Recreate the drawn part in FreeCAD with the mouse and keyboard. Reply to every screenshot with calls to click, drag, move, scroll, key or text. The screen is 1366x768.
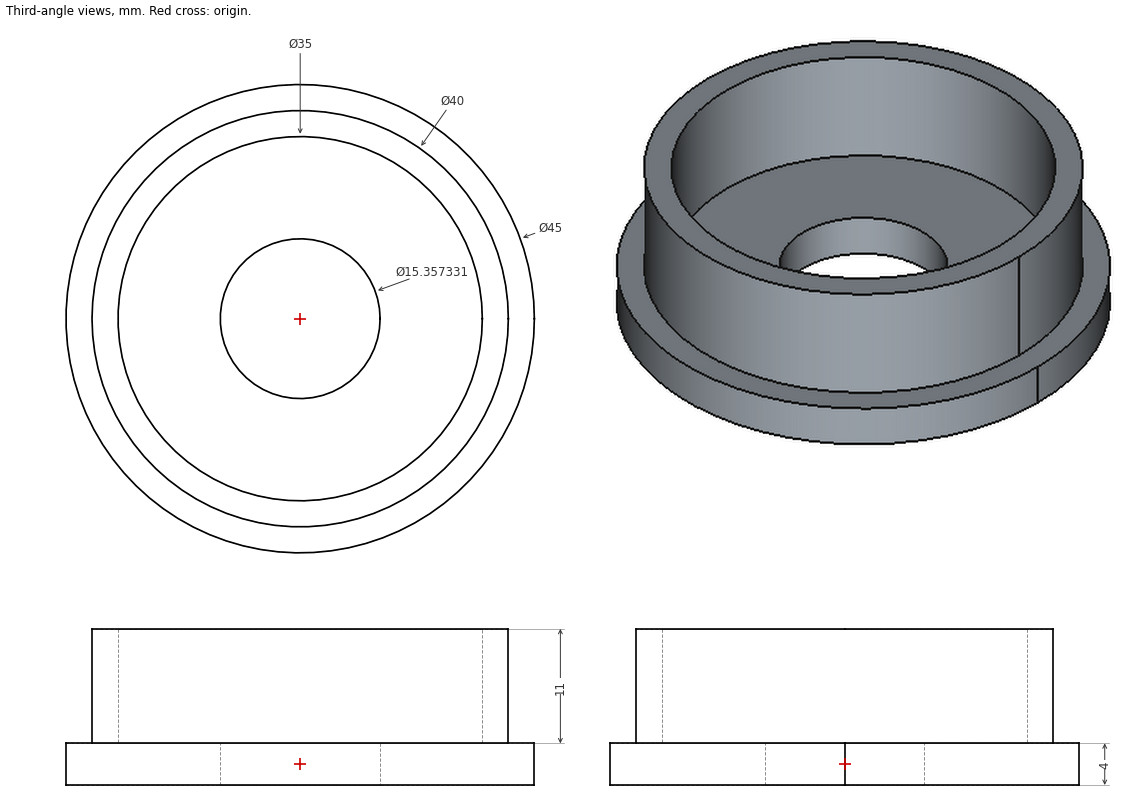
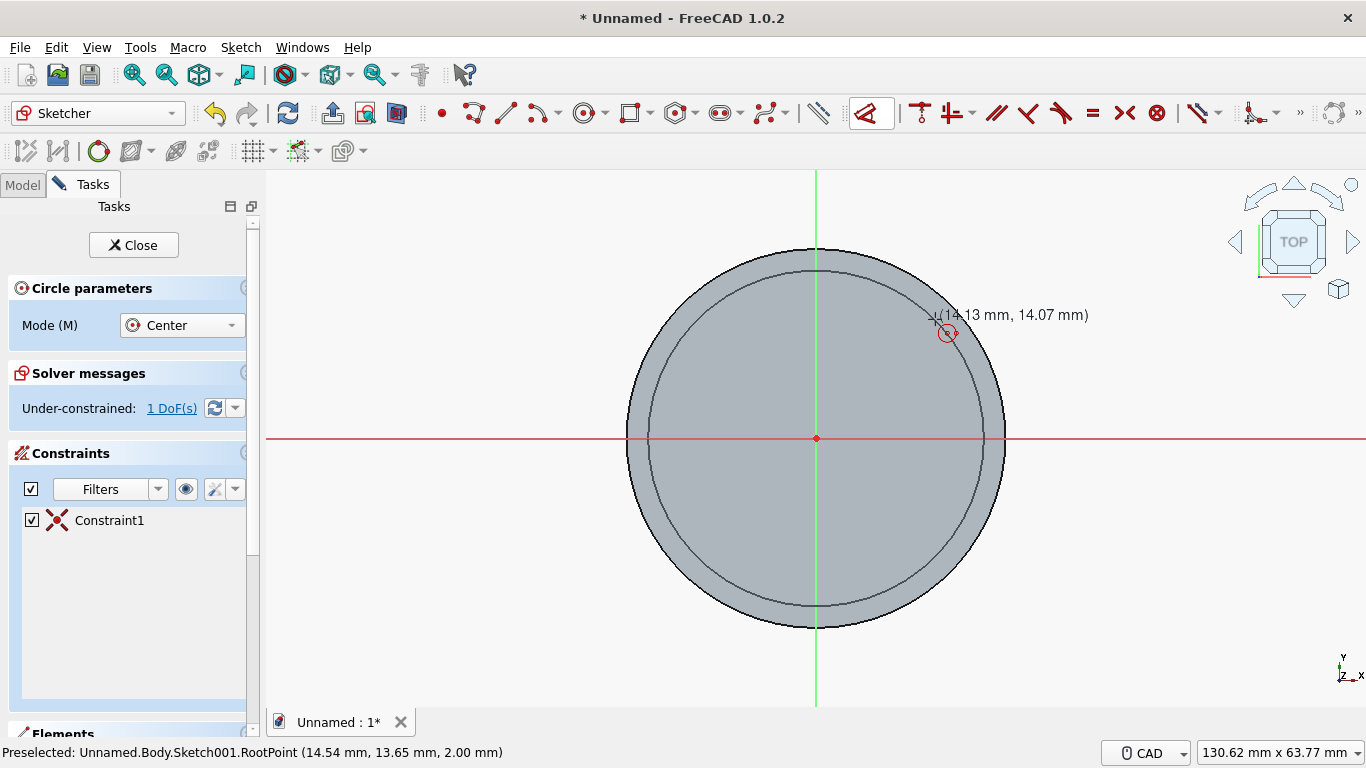
click(816, 438)
click(920, 334)
key(Escape)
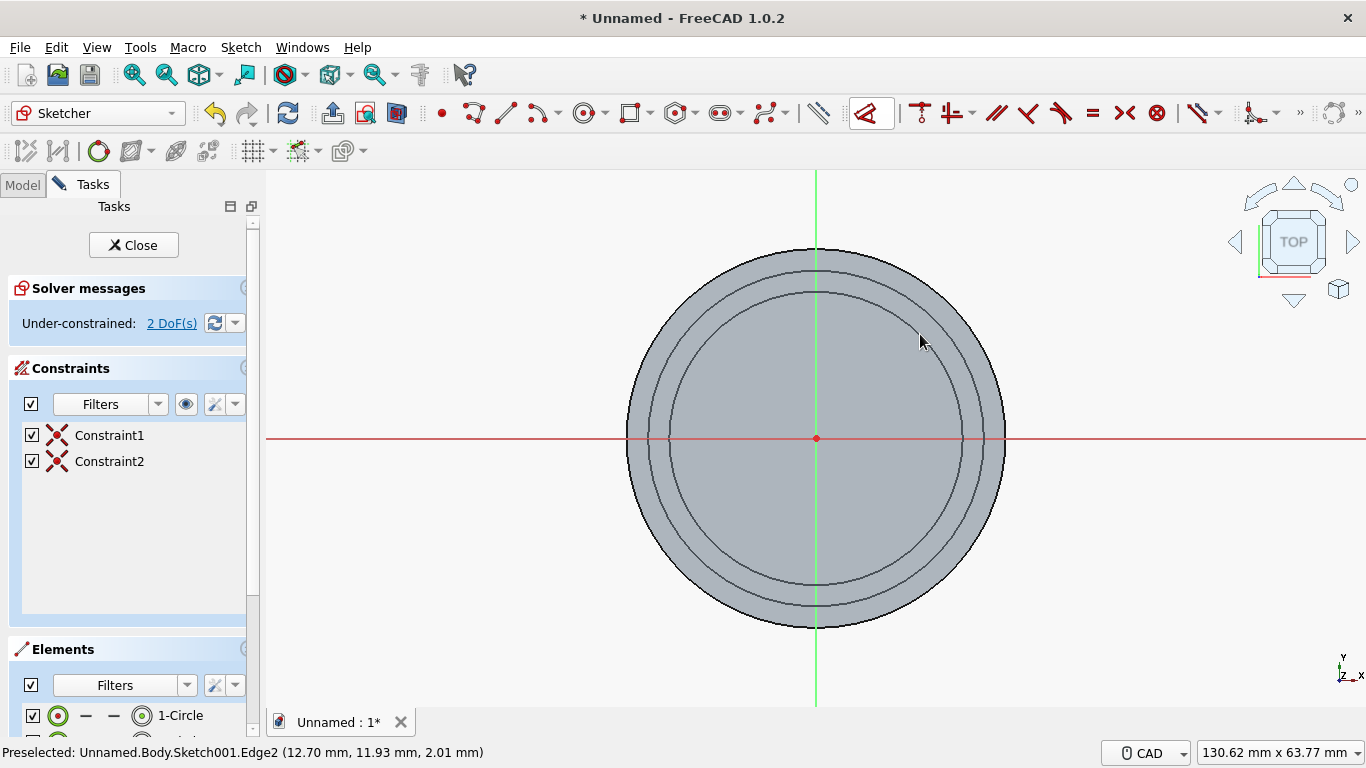
click(866, 114)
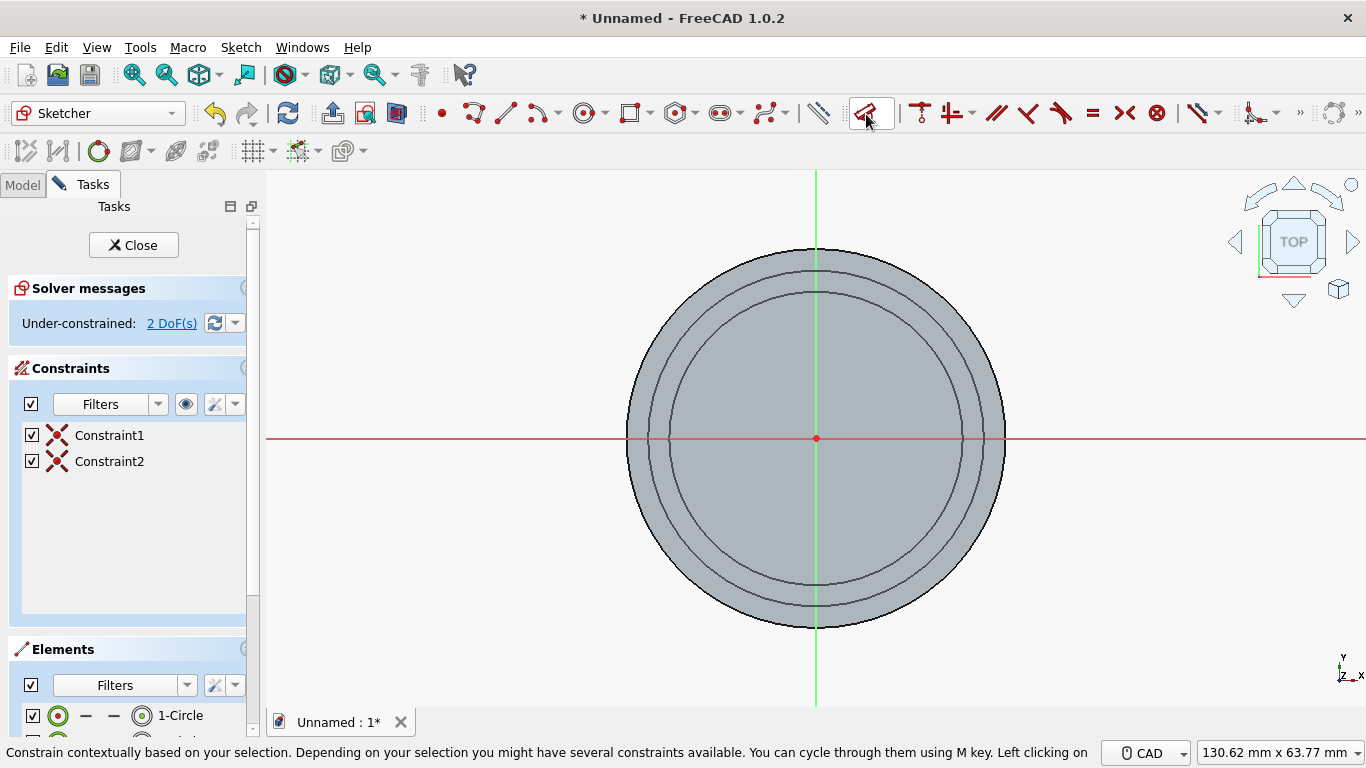
click(934, 319)
click(956, 296)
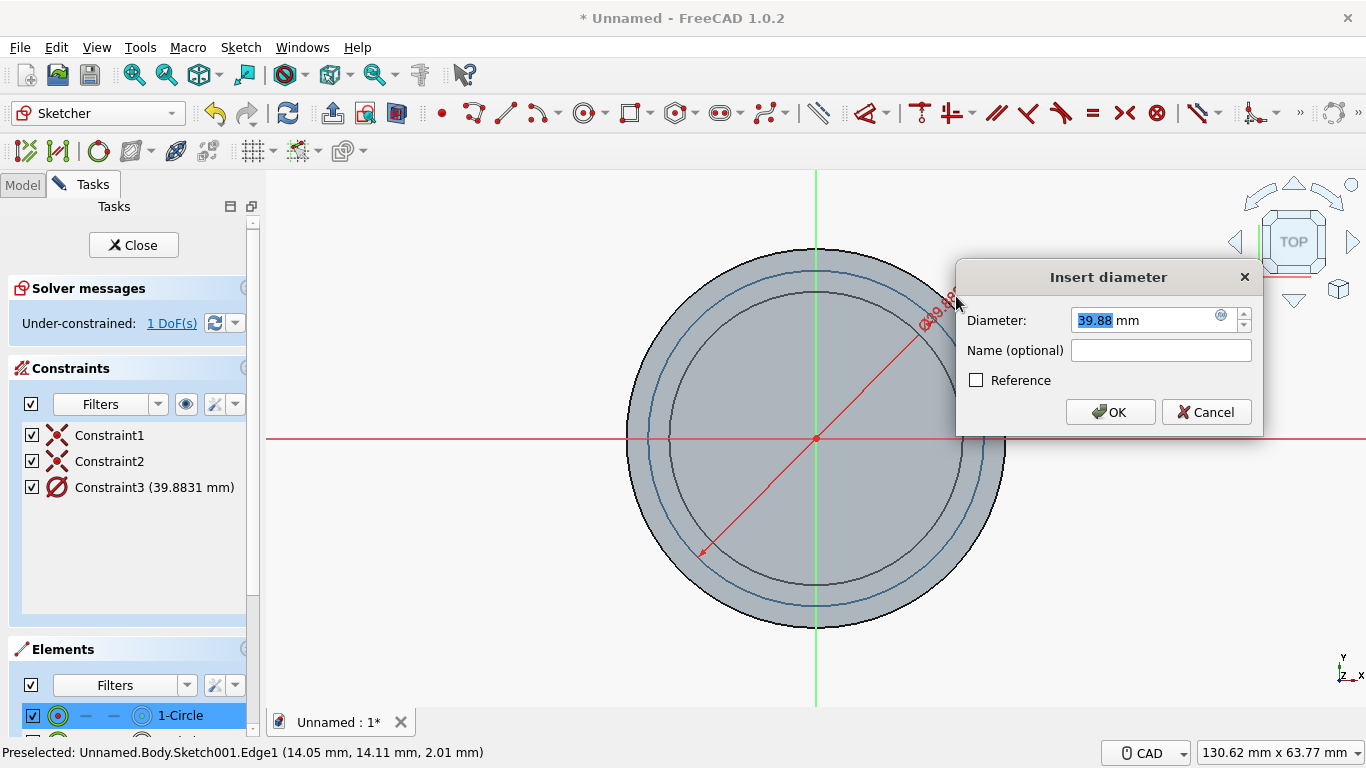
text(40)
key(Return)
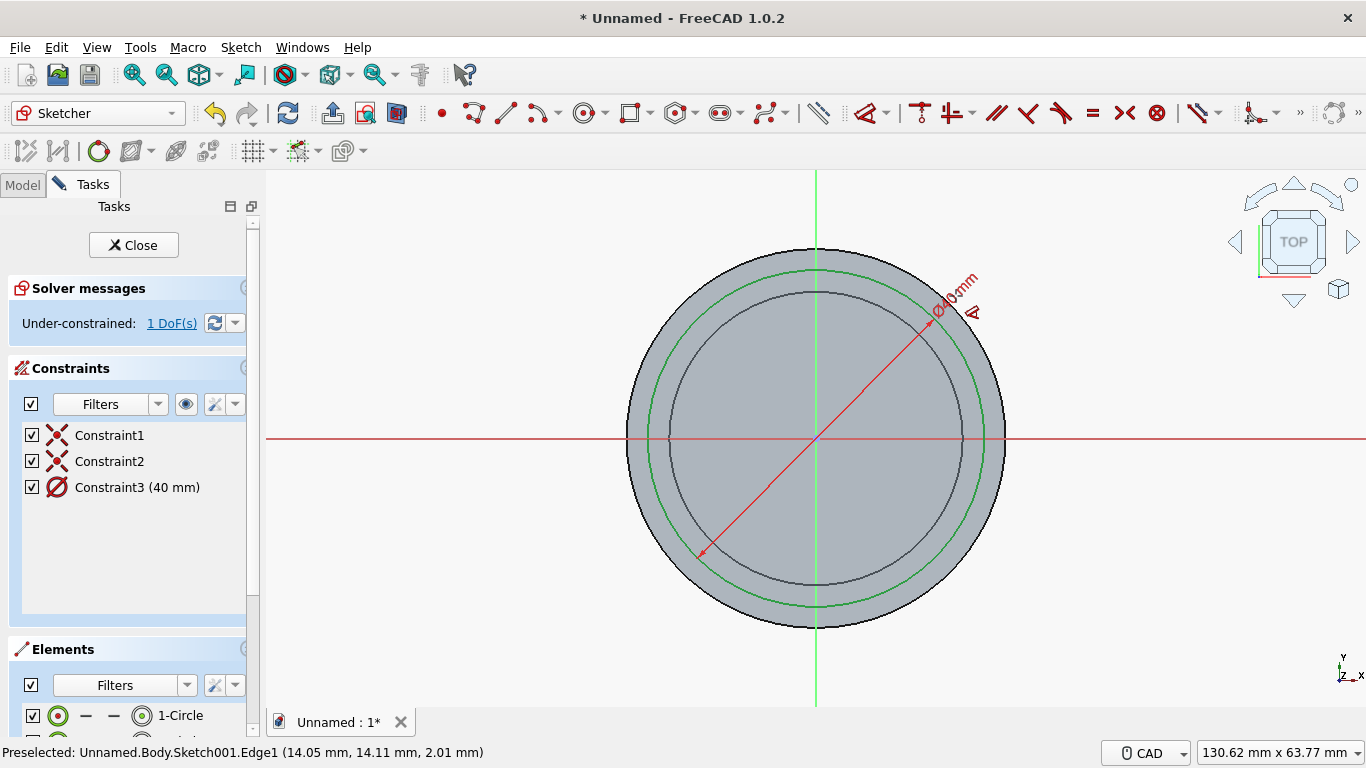
click(919, 334)
click(1009, 380)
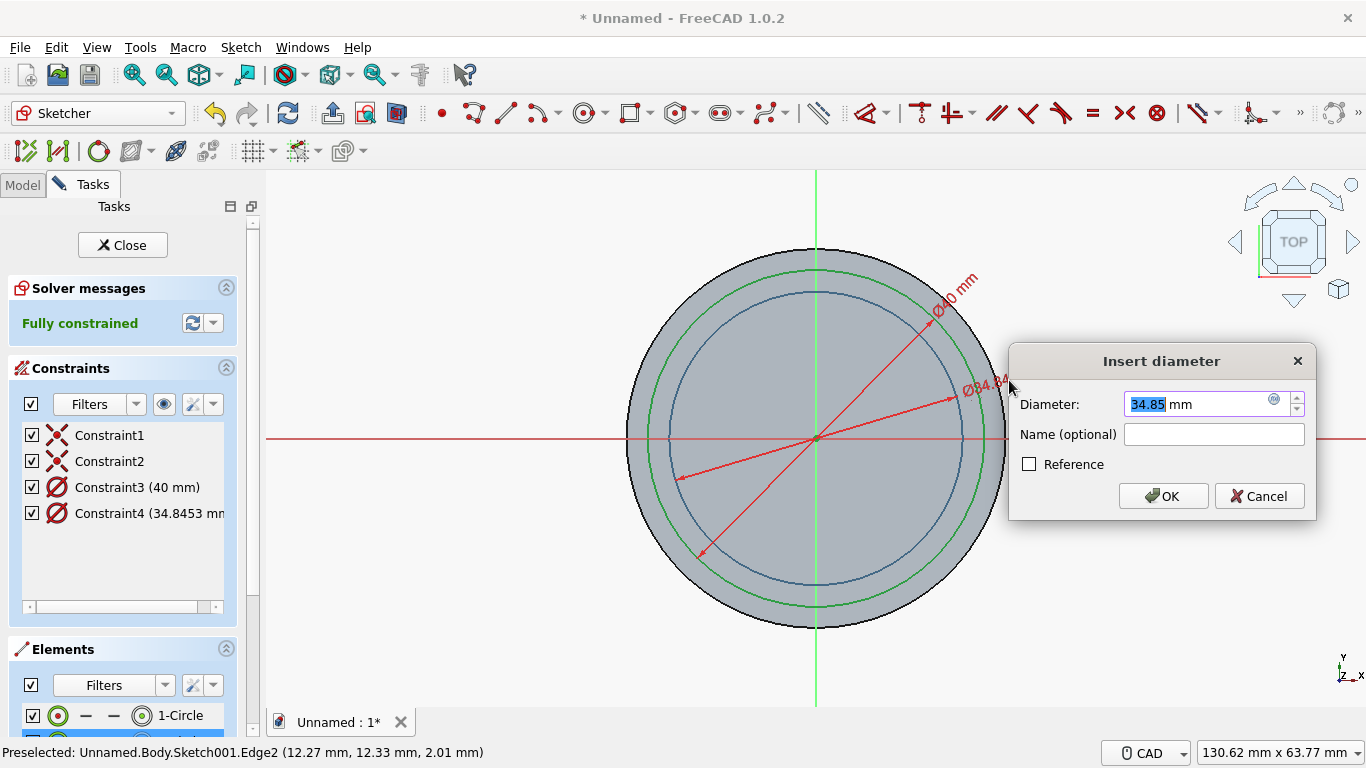
text(35)
key(Return)
key(Escape)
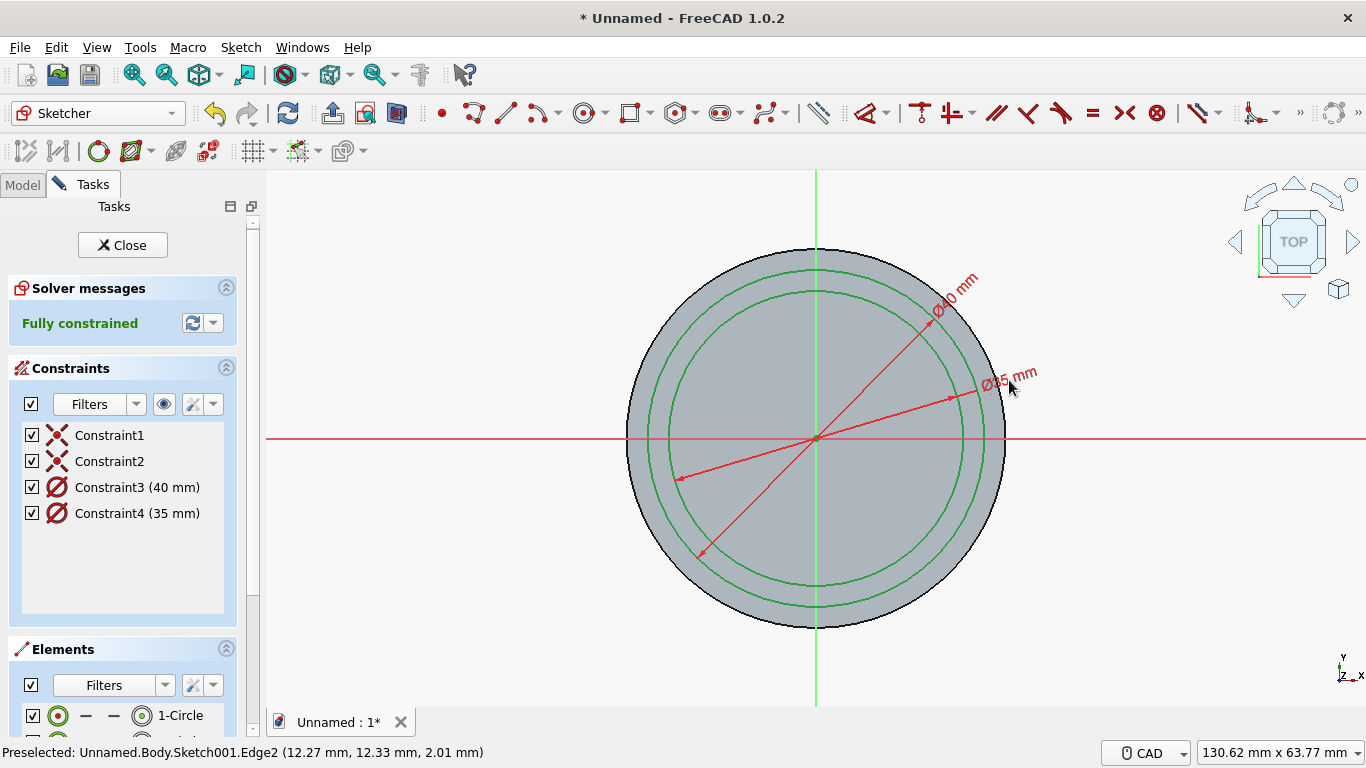
click(123, 245)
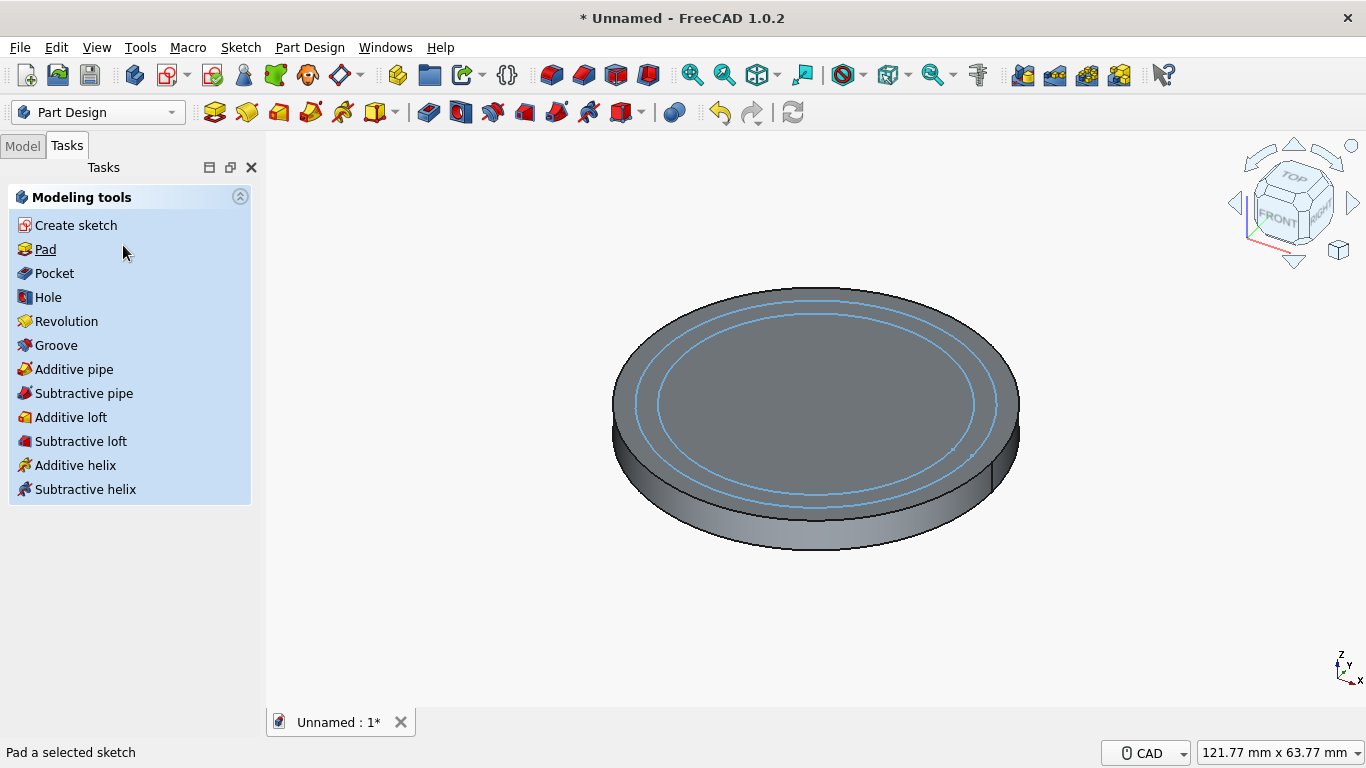
click(216, 112)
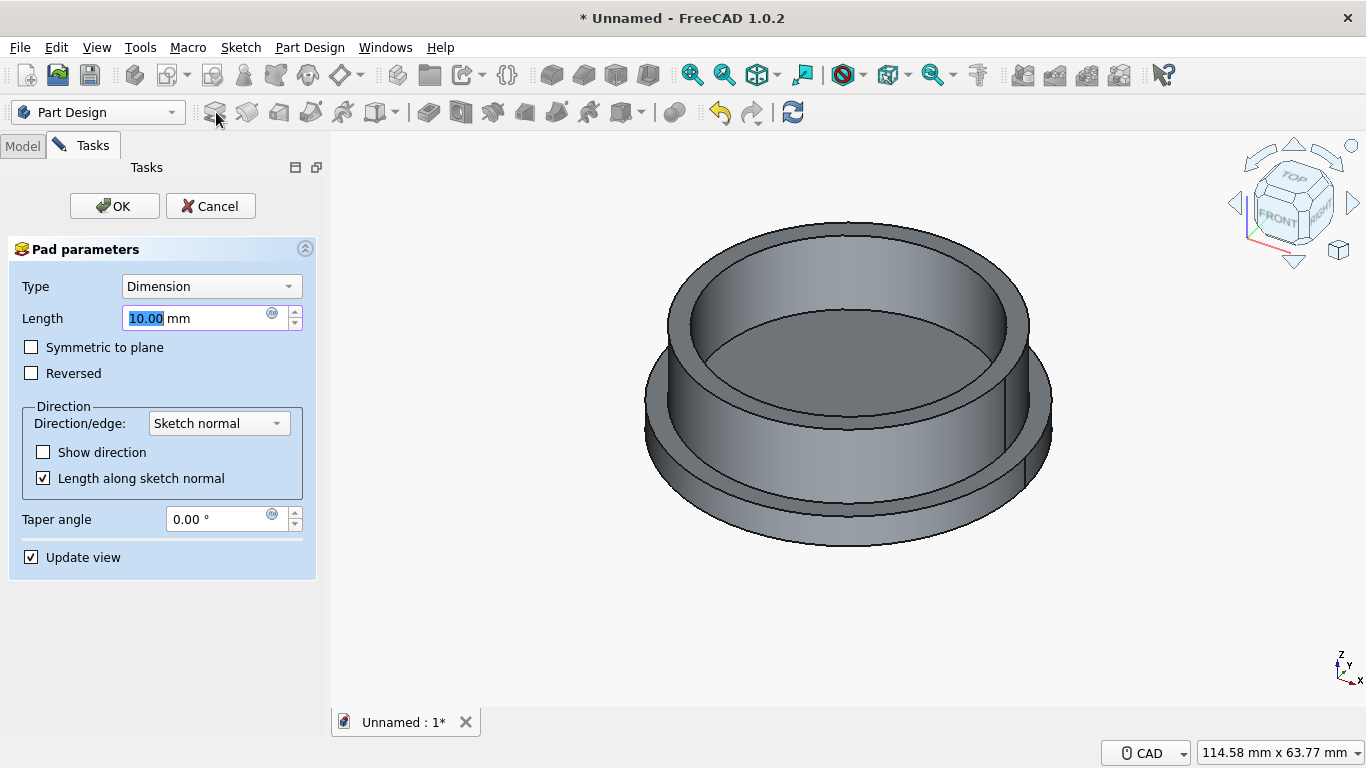
text(11)
key(Tab)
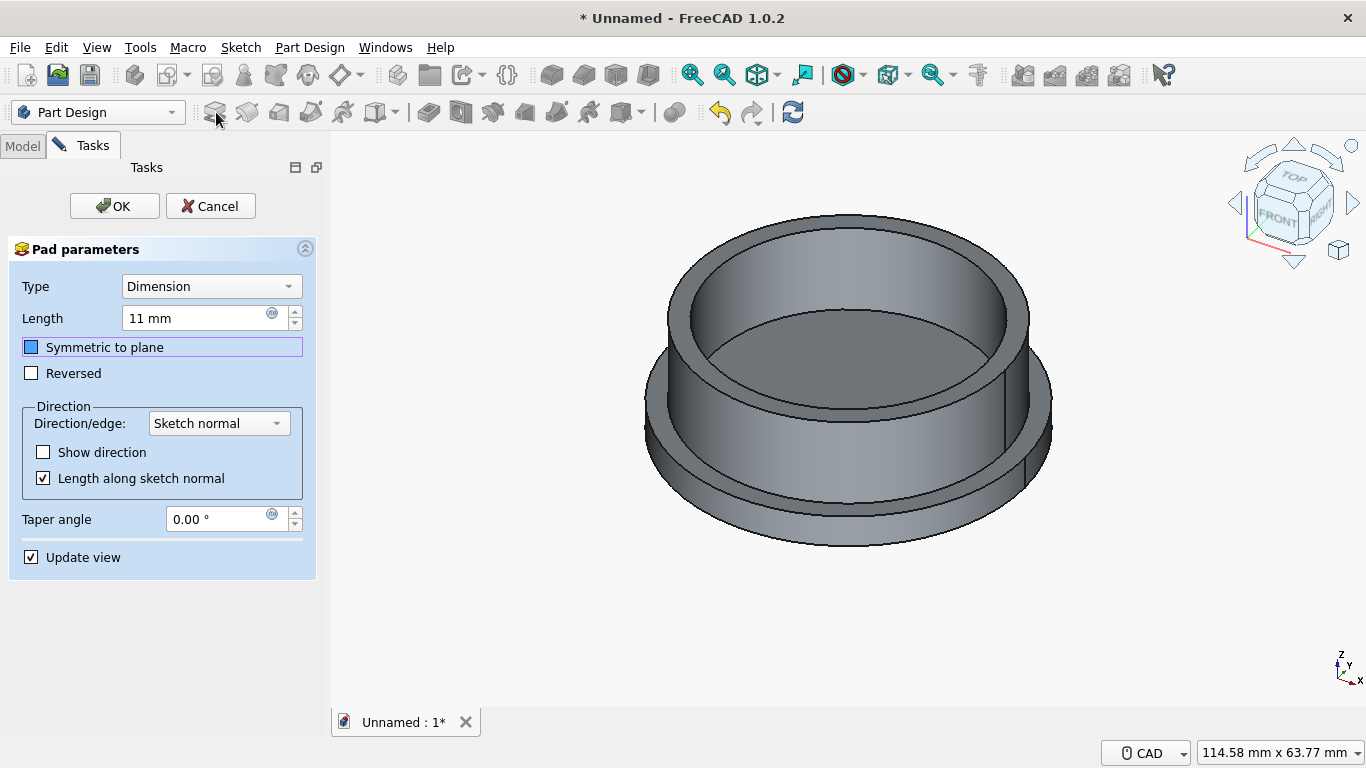
click(115, 206)